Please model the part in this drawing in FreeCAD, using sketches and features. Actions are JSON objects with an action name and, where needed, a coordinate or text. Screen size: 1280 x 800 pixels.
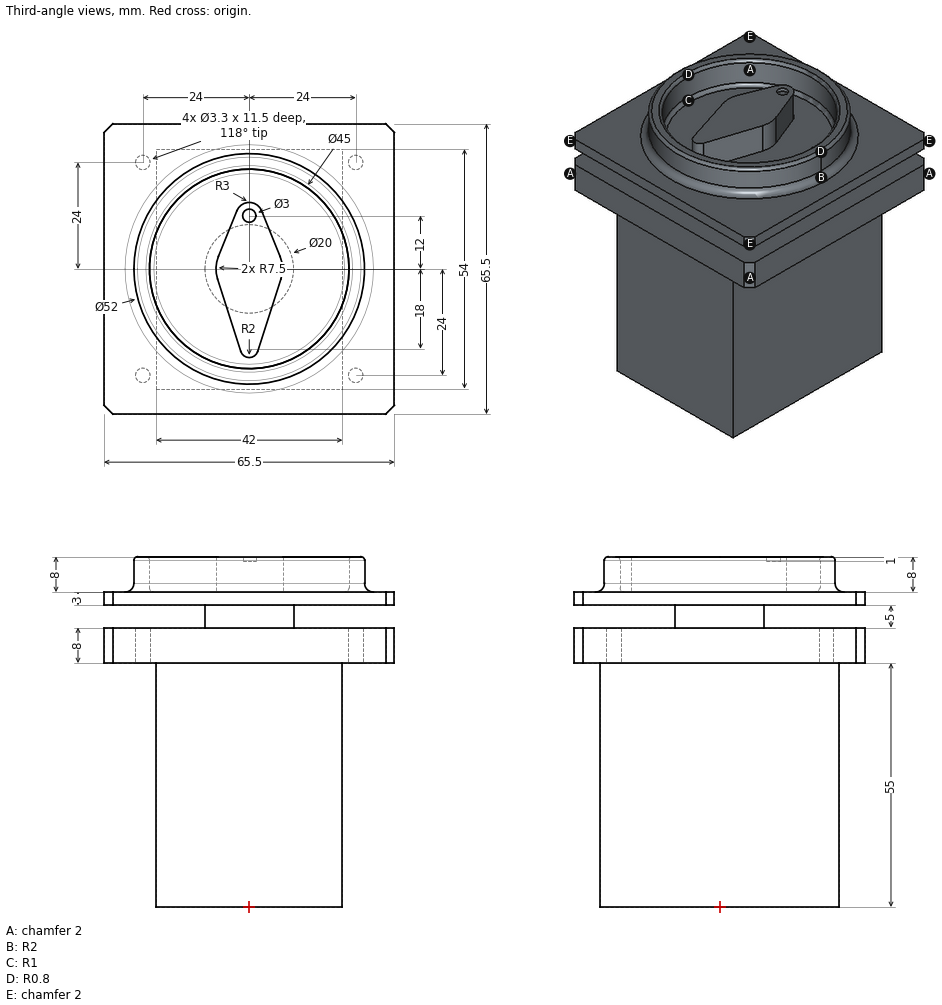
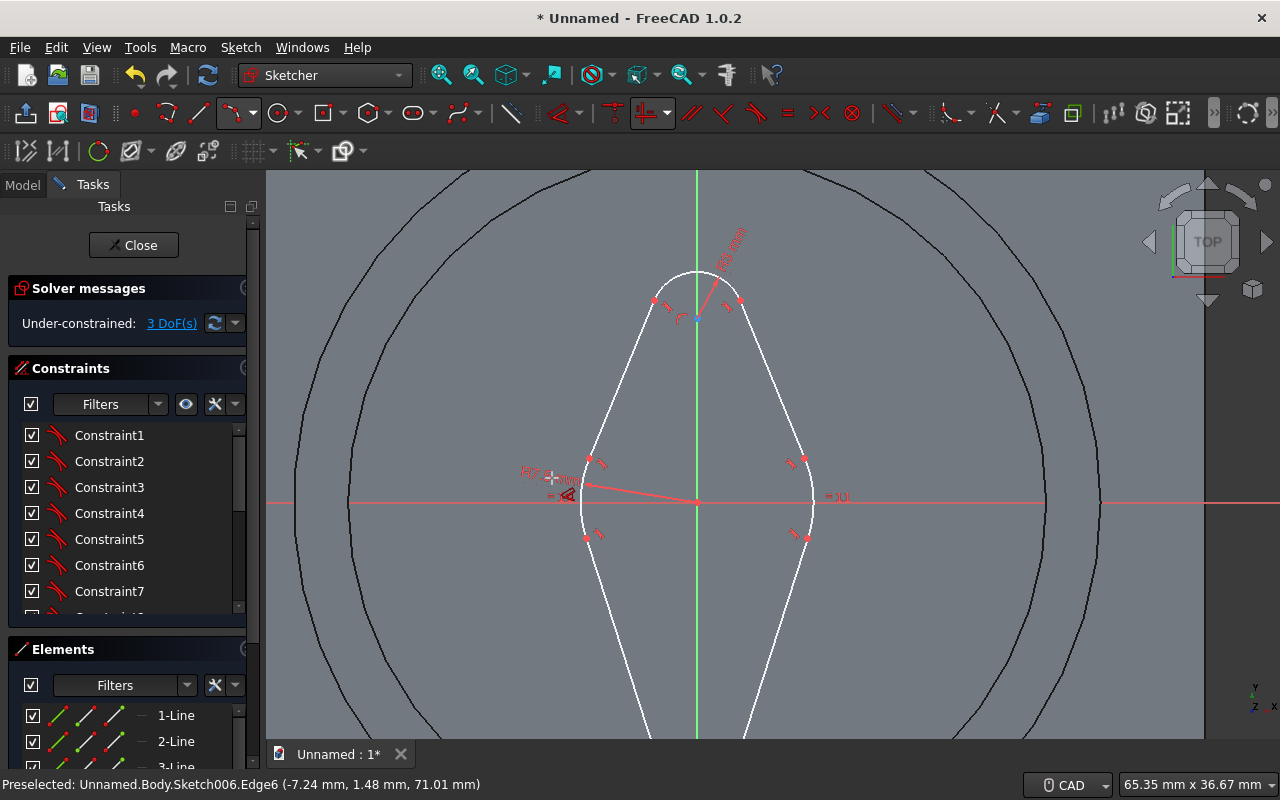
{"action": "scroll", "coordinate": [719, 278], "scroll_direction": "down", "scroll_amount": 2}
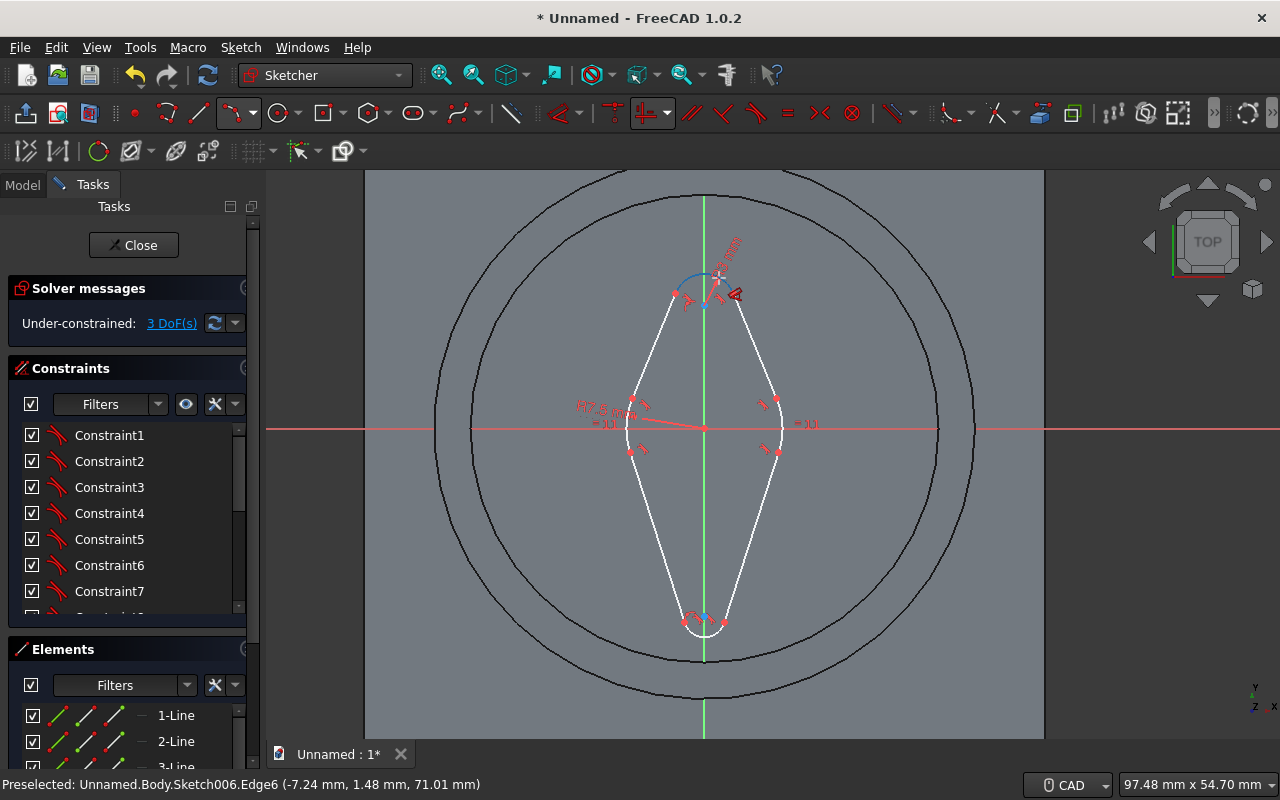
{"action": "scroll", "coordinate": [695, 635], "scroll_direction": "up", "scroll_amount": 4}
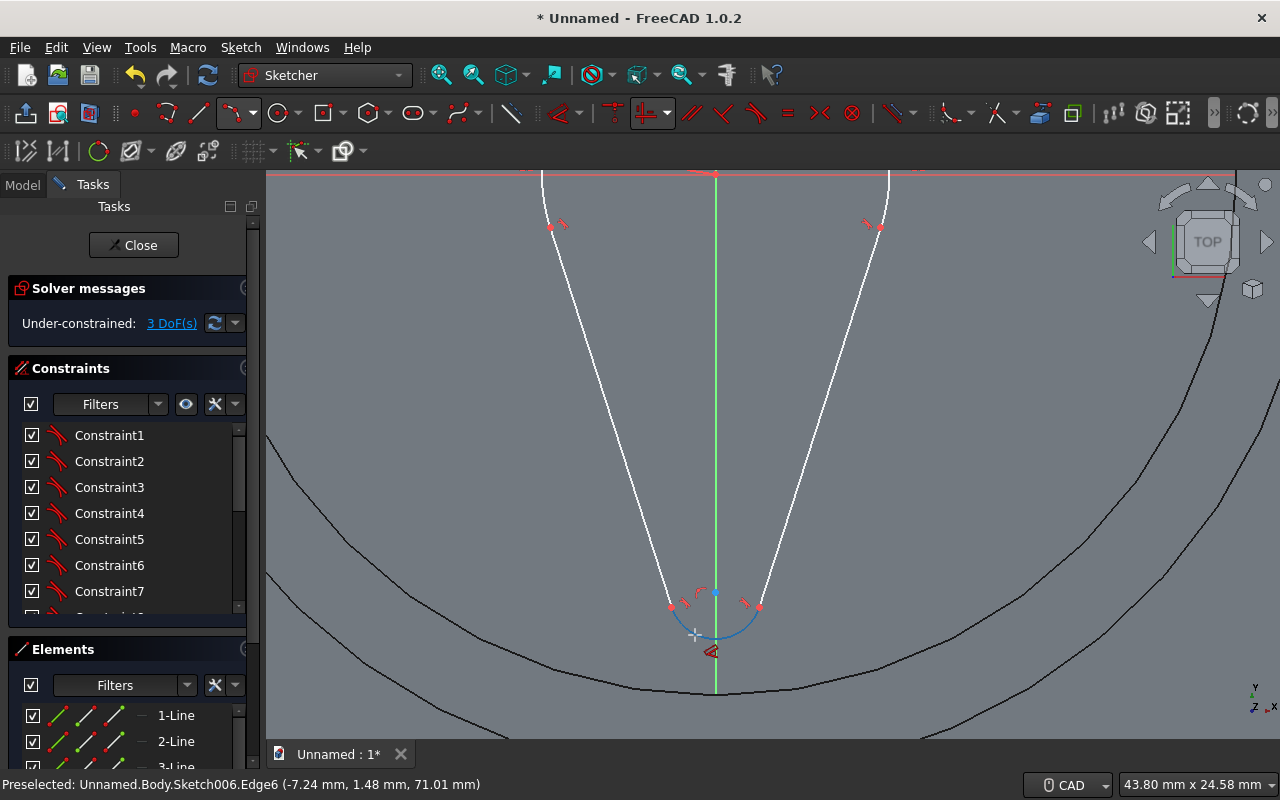
{"action": "left_click", "coordinate": [693, 633]}
{"action": "left_click", "coordinate": [677, 661]}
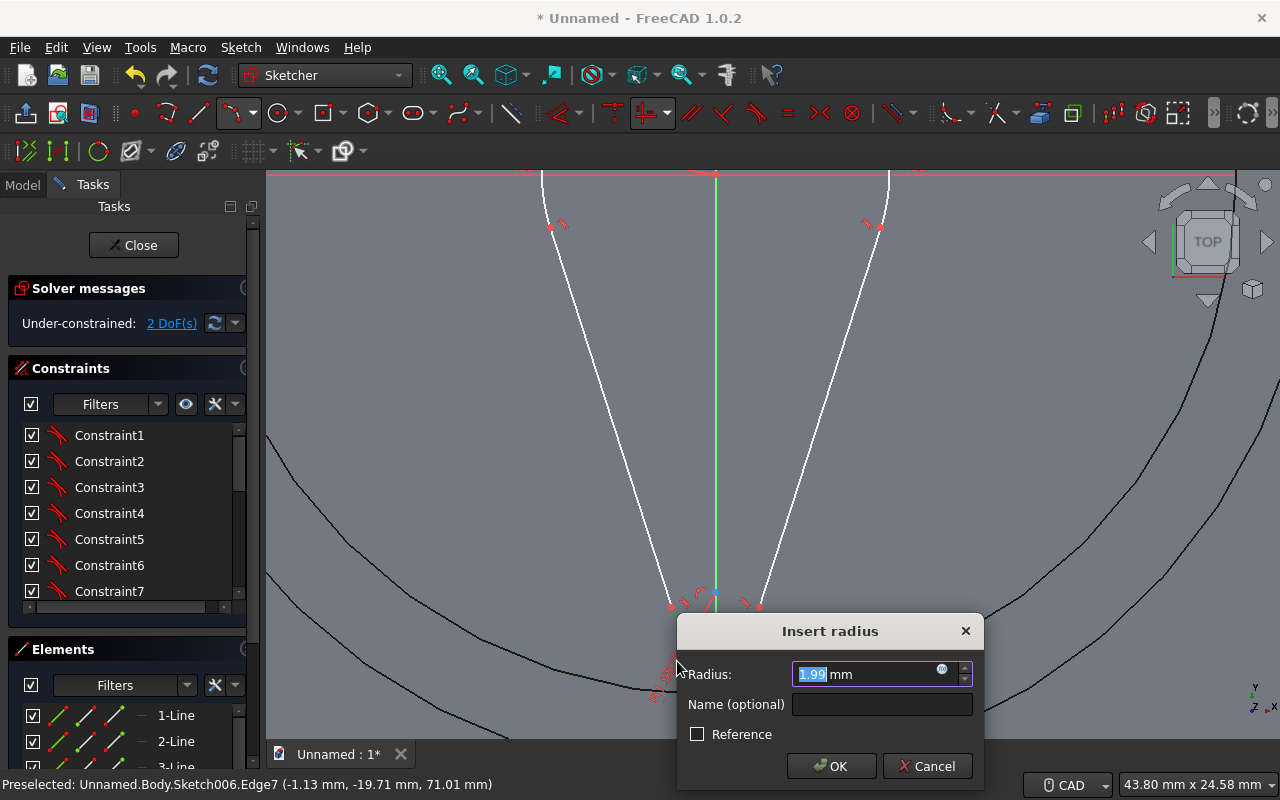
{"action": "type", "text": "2"}
{"action": "key", "text": "Return"}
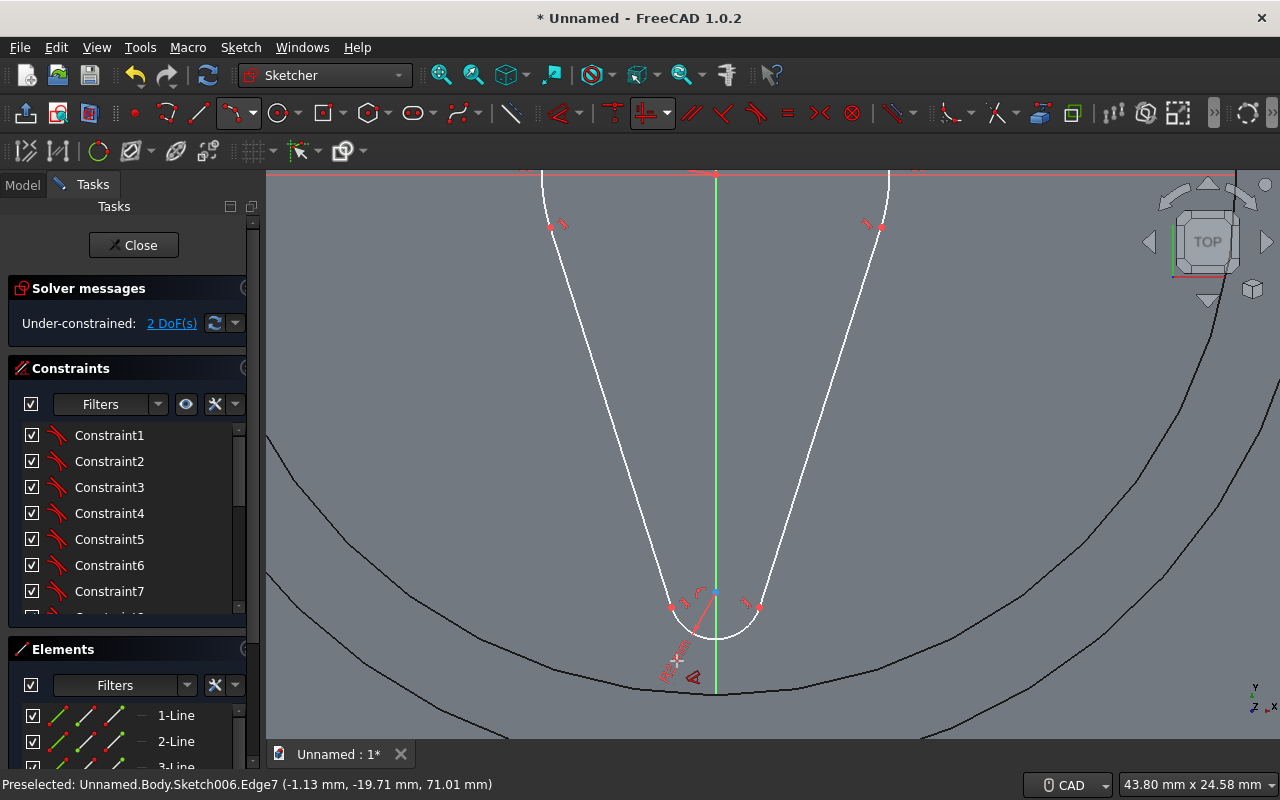
{"action": "scroll", "coordinate": [695, 636], "scroll_direction": "down", "scroll_amount": 4}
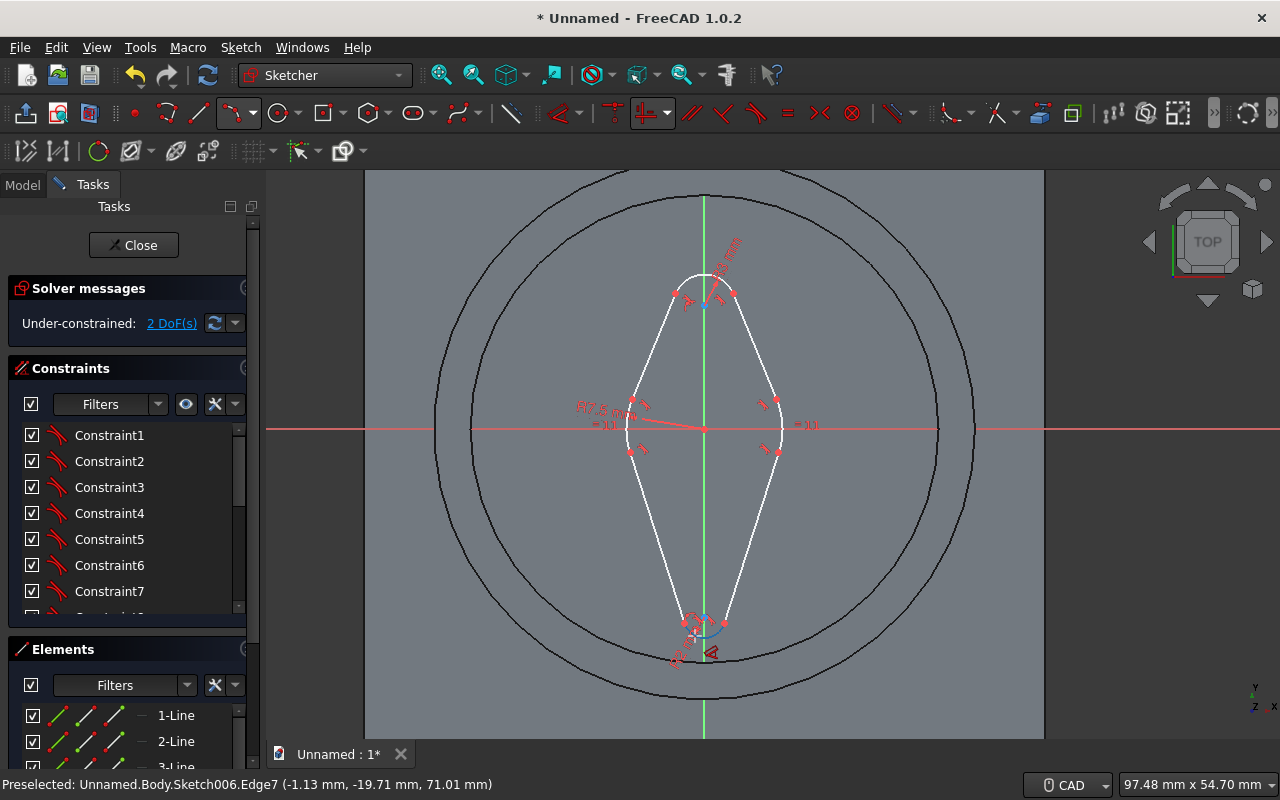
{"action": "left_click", "coordinate": [704, 306]}
{"action": "left_click", "coordinate": [738, 367]}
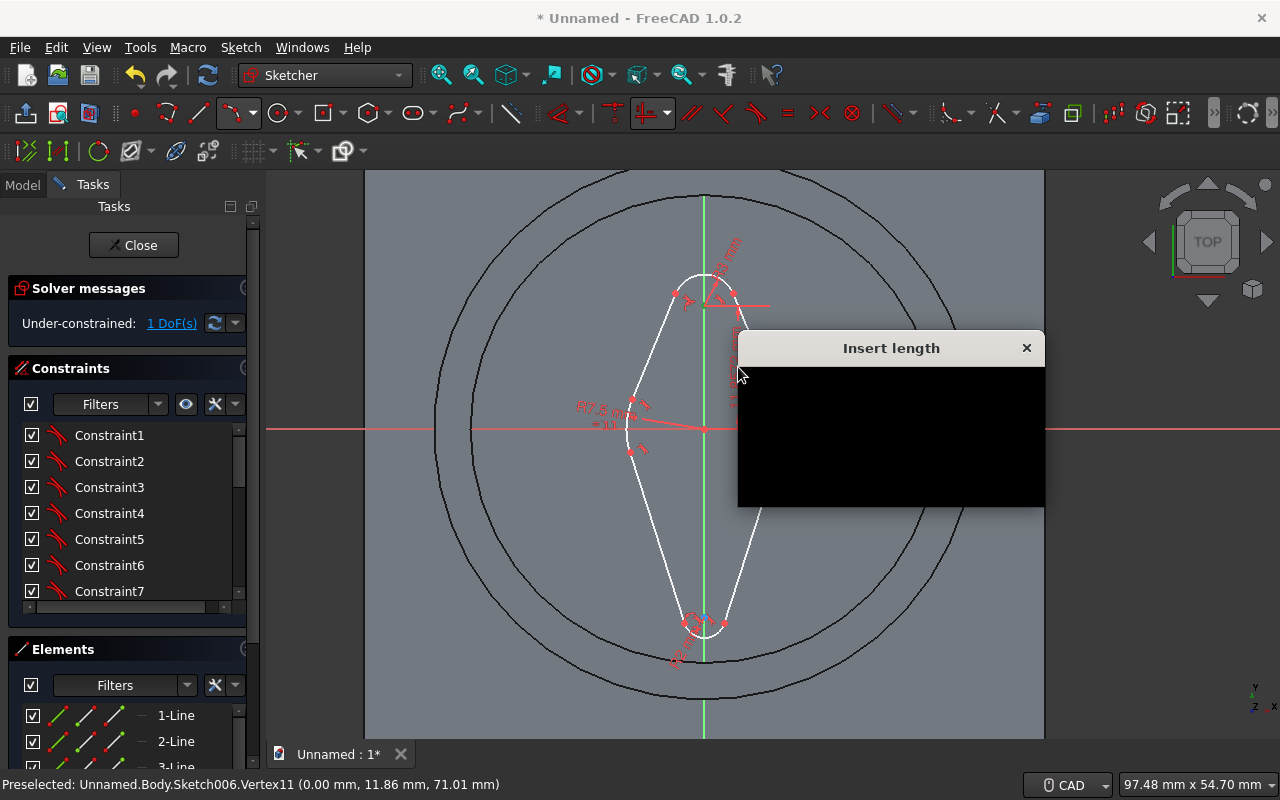
{"action": "type", "text": "12"}
{"action": "key", "text": "Return"}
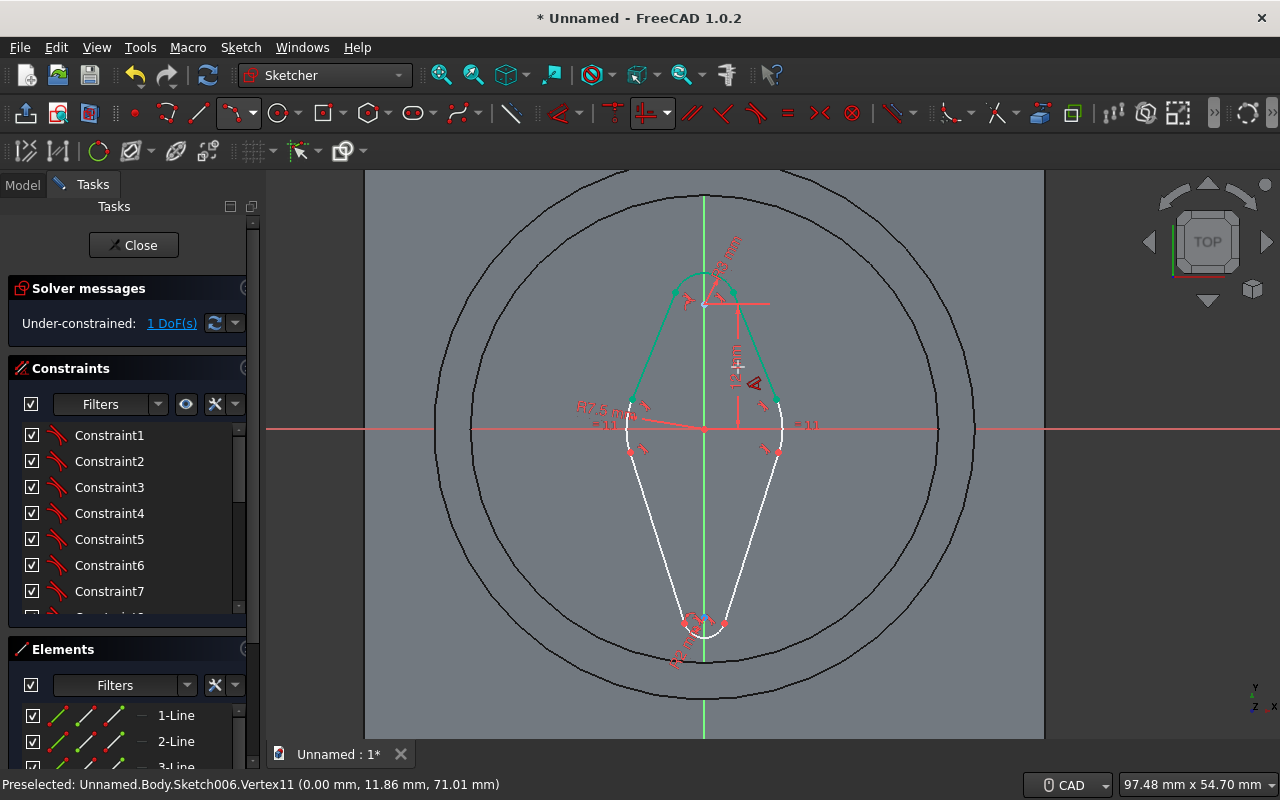
{"action": "left_click", "coordinate": [704, 617]}
{"action": "left_click", "coordinate": [738, 523]}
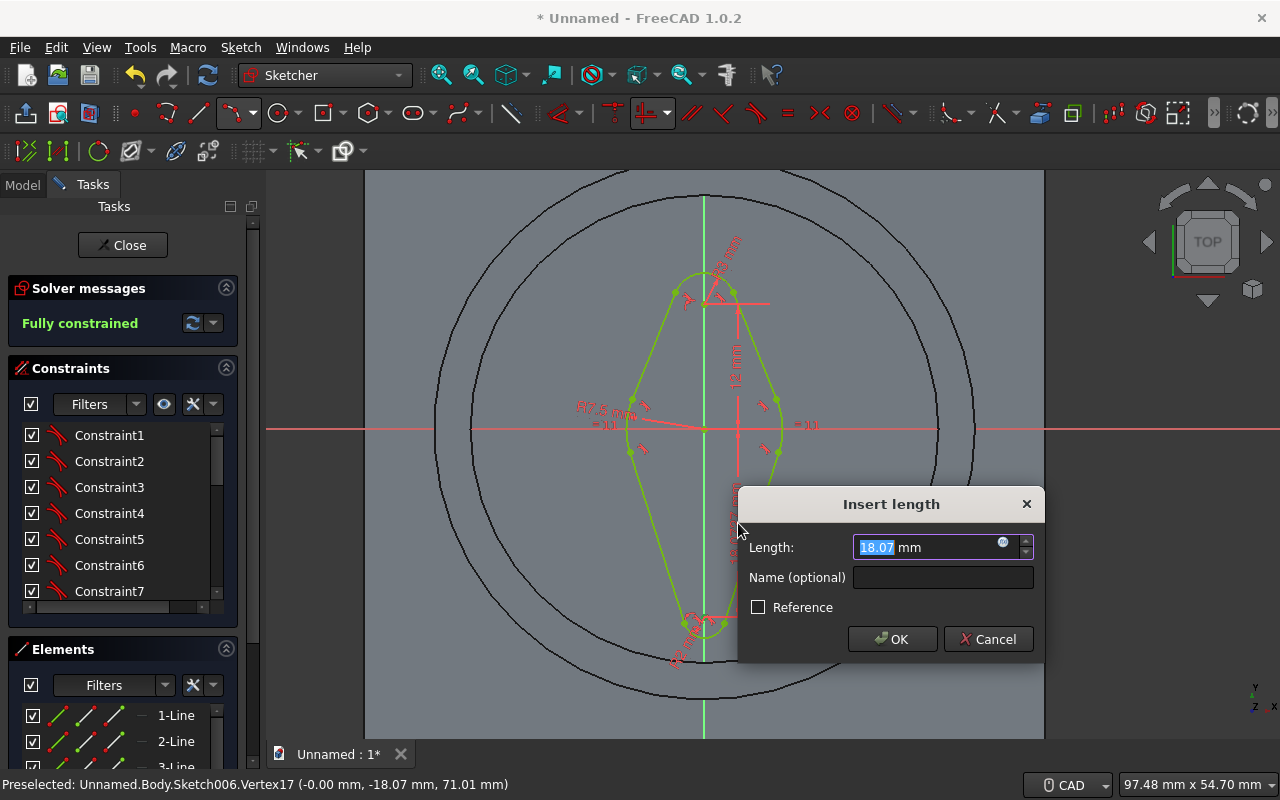
{"action": "type", "text": "18"}
{"action": "key", "text": "Return"}
{"action": "key", "text": "Escape"}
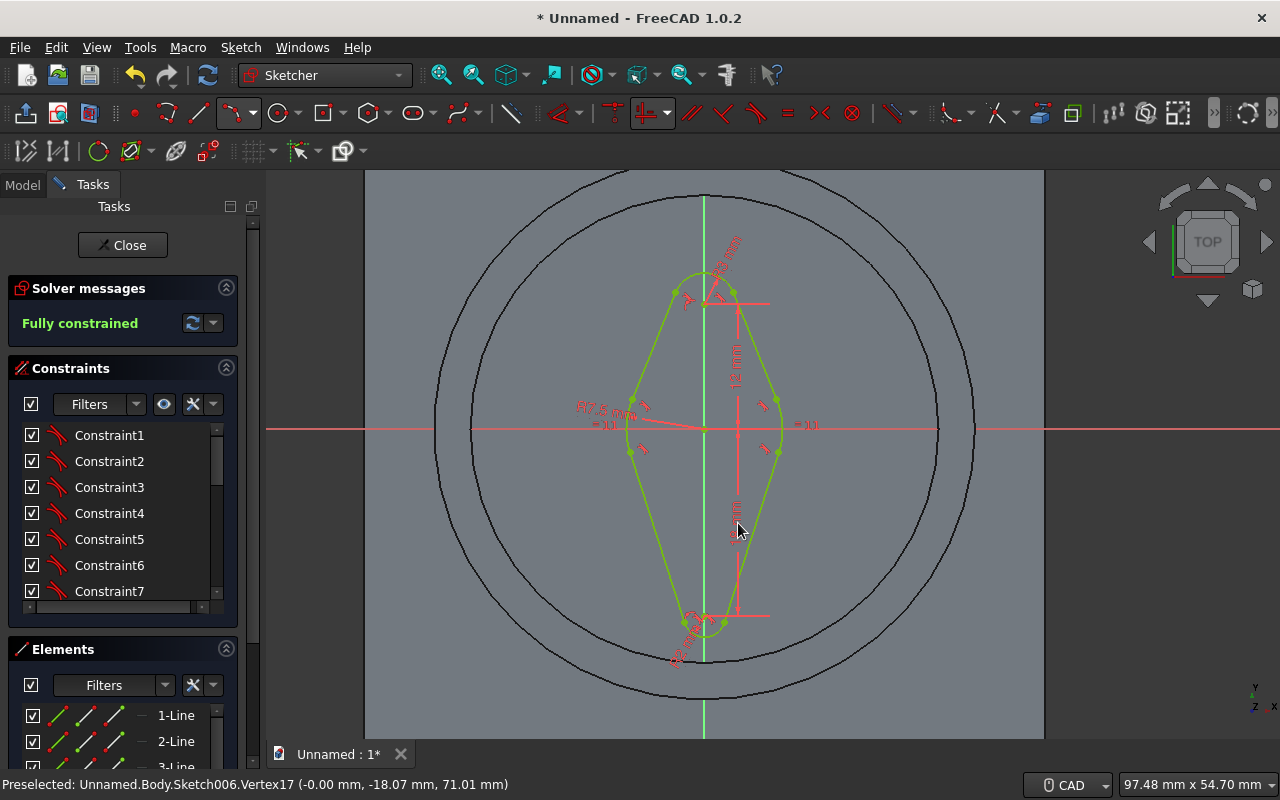
{"action": "left_click", "coordinate": [123, 245]}